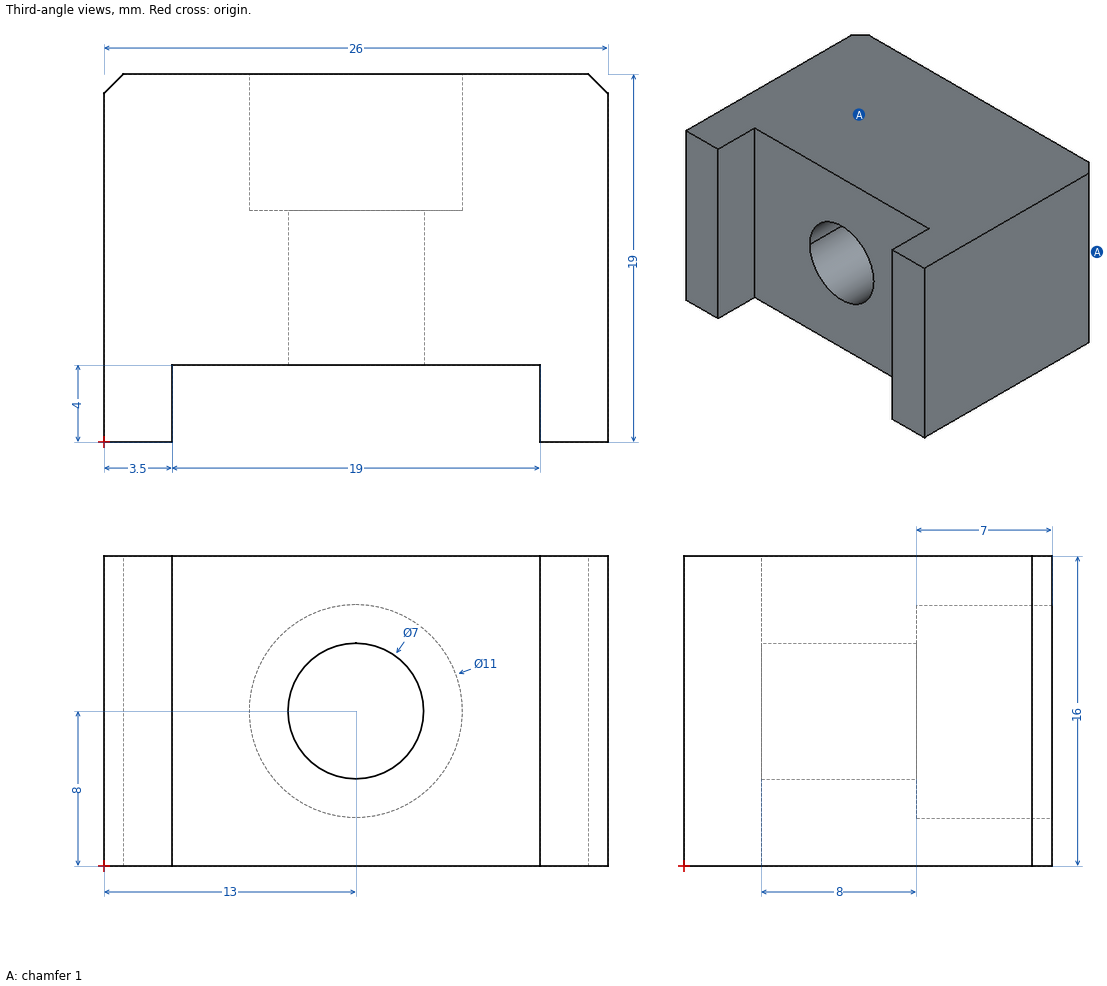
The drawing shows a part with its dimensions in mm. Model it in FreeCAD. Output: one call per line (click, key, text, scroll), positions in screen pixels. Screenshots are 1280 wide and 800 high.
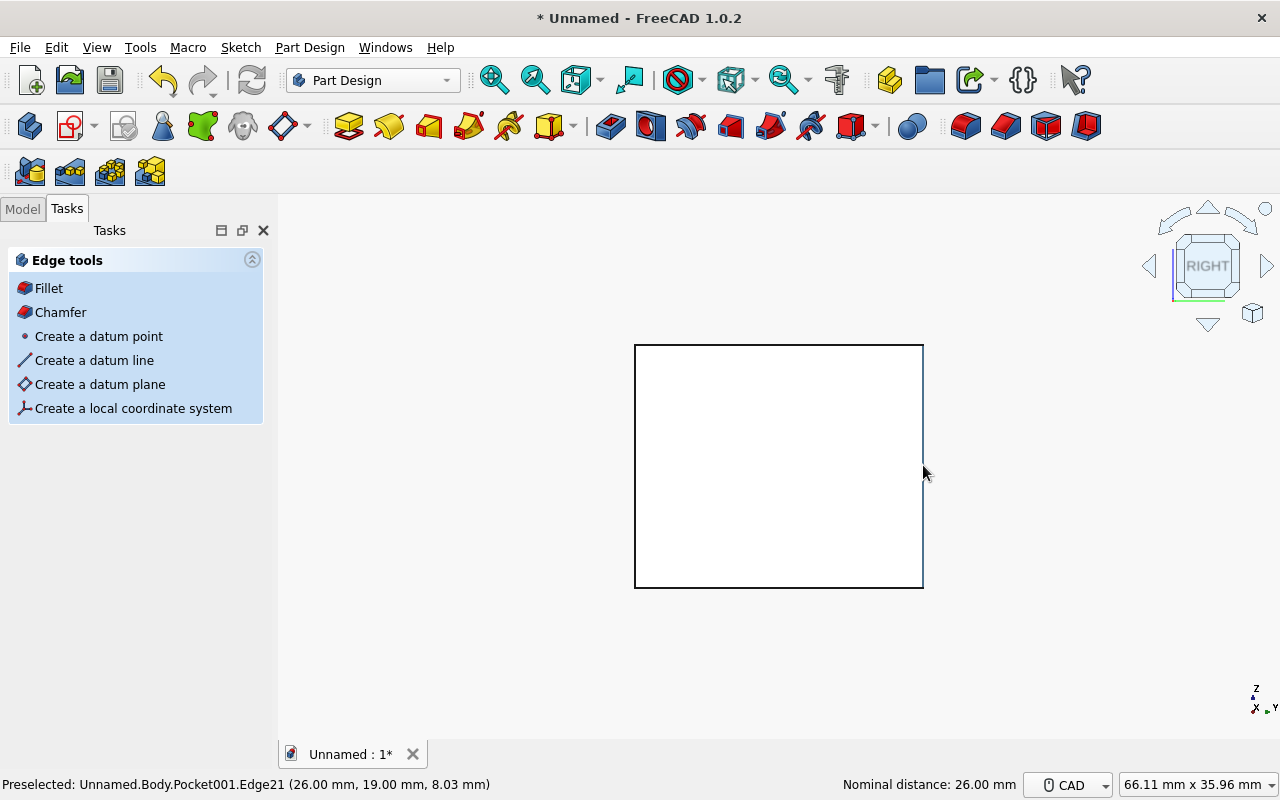
click(1006, 126)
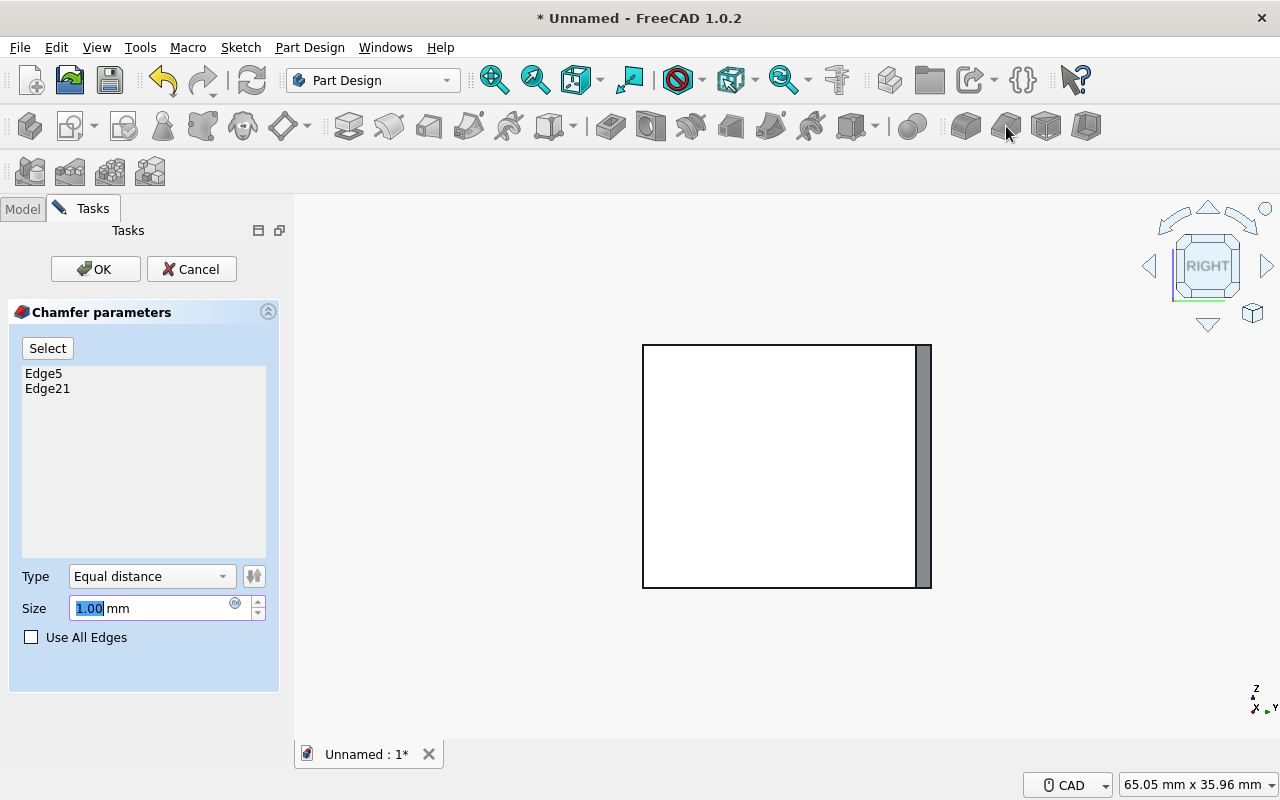
text(1)
key(Tab)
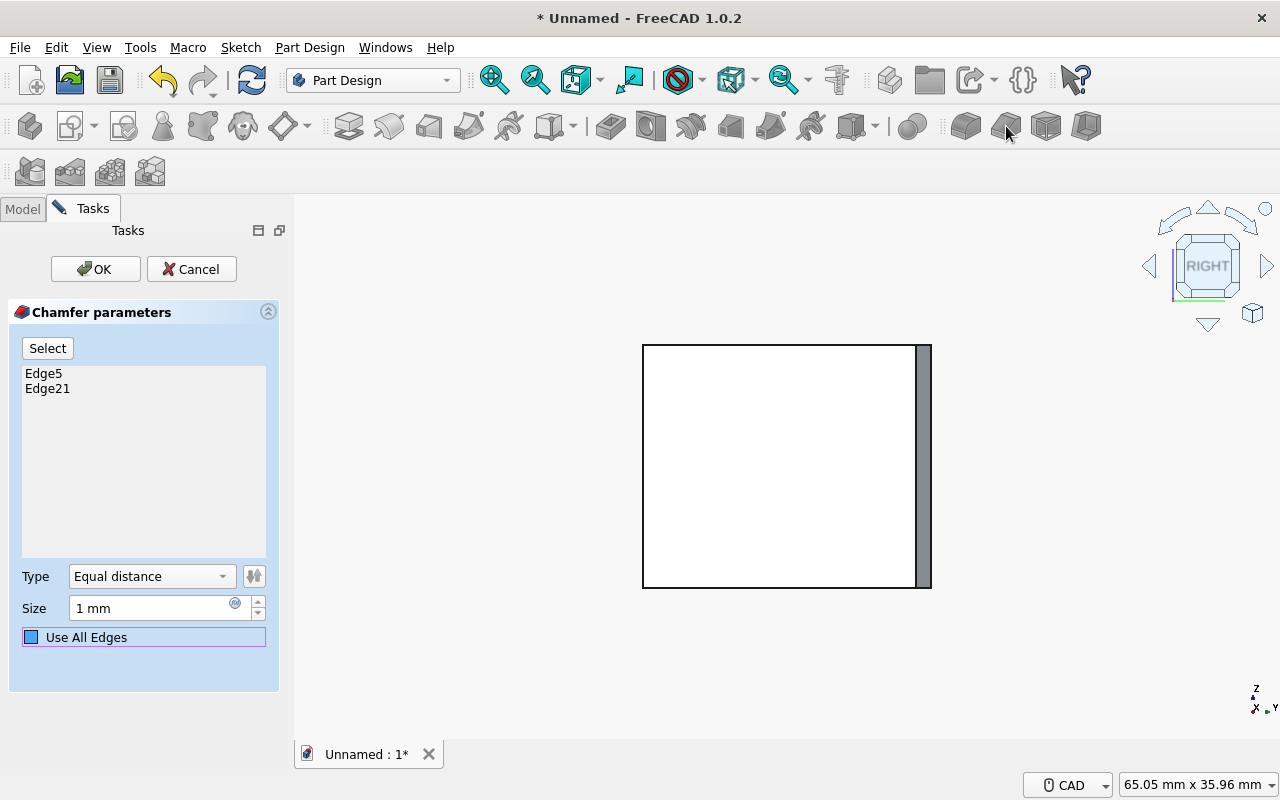
click(96, 269)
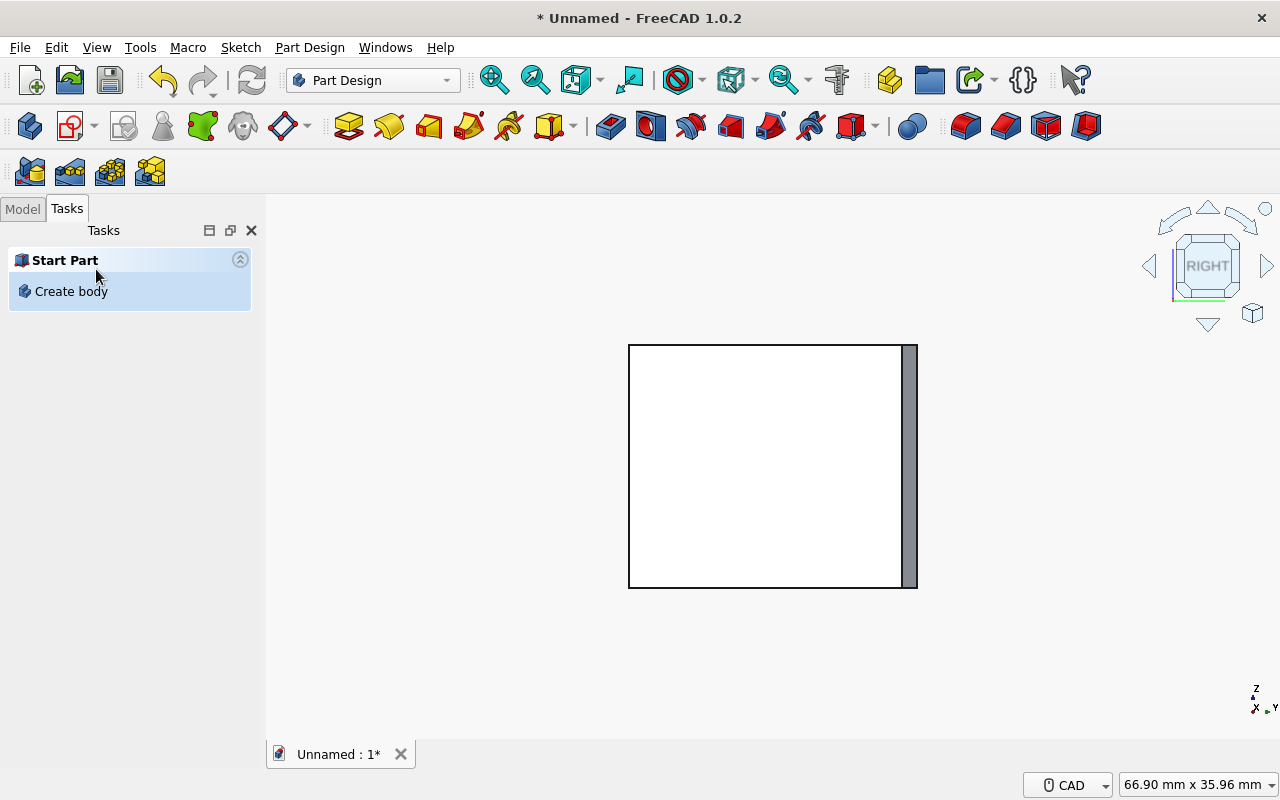
key(0)